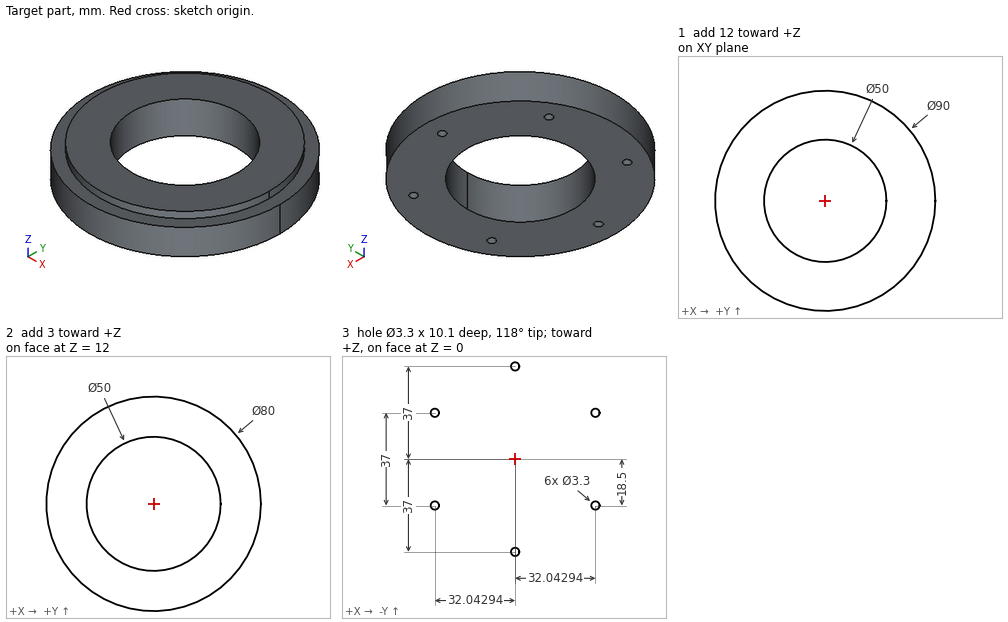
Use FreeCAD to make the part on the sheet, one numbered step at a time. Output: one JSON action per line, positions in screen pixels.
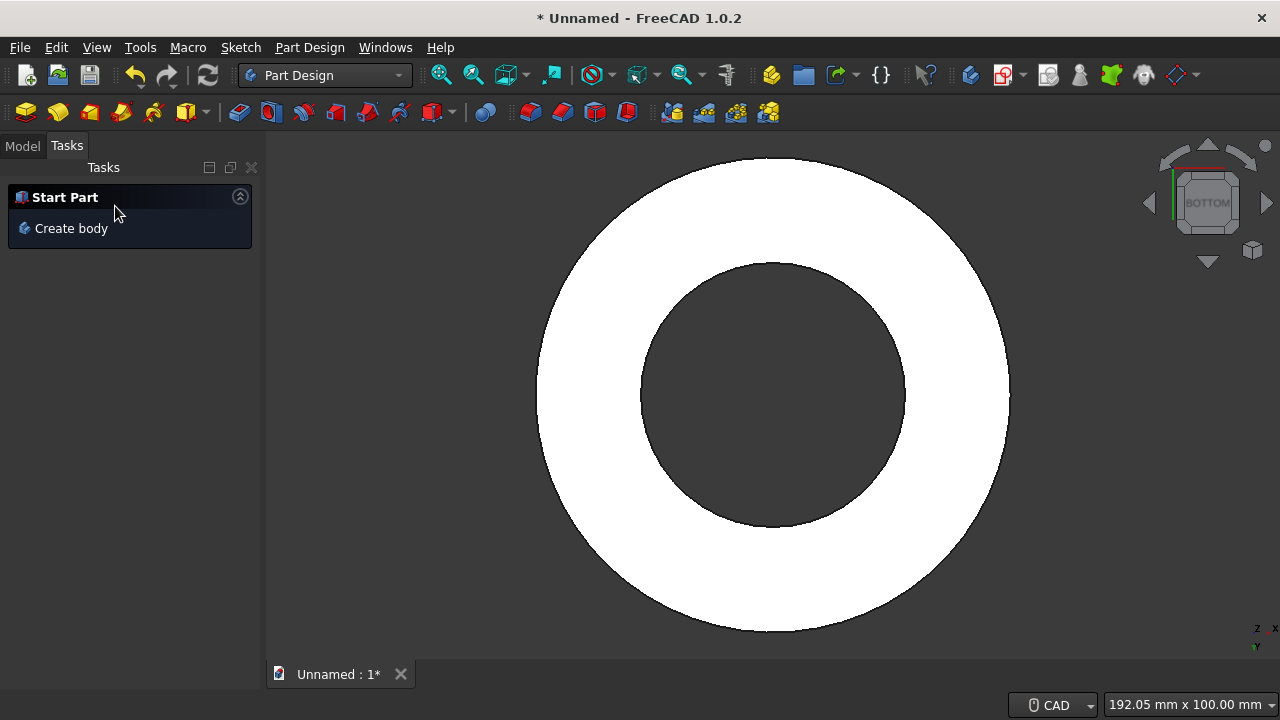
{"action": "left_click", "coordinate": [909, 530]}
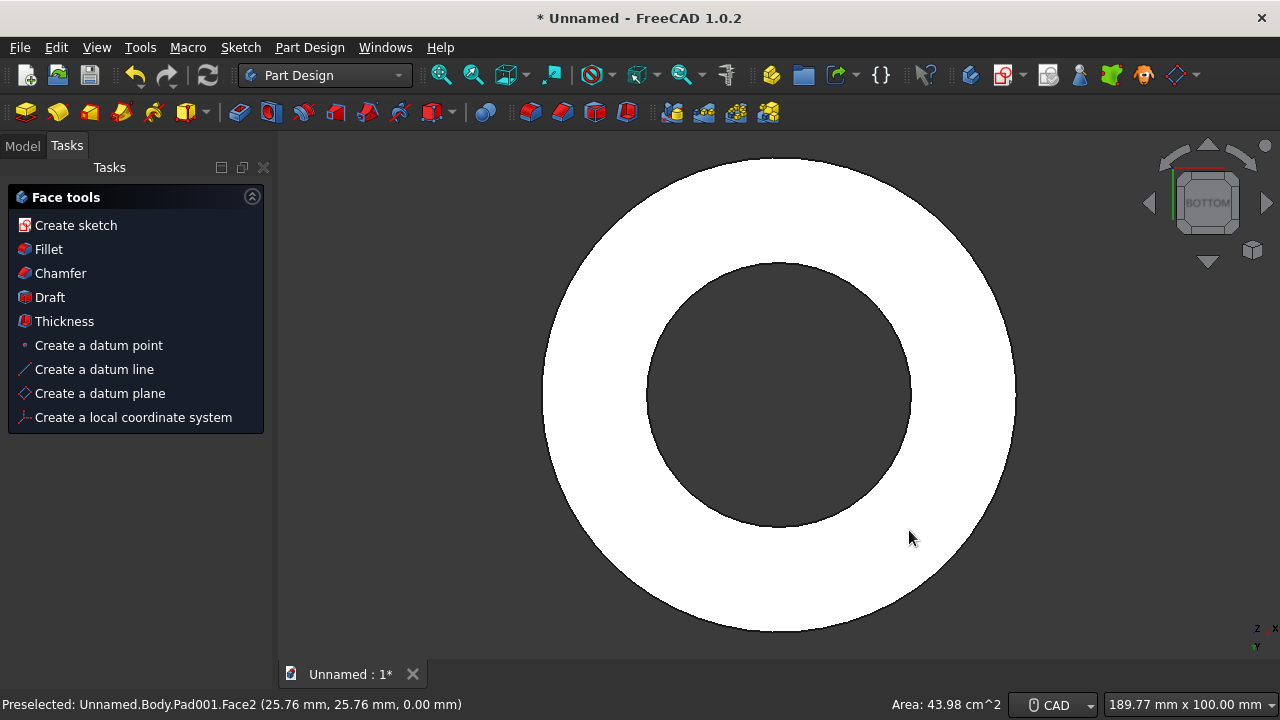
{"action": "left_click", "coordinate": [1004, 76]}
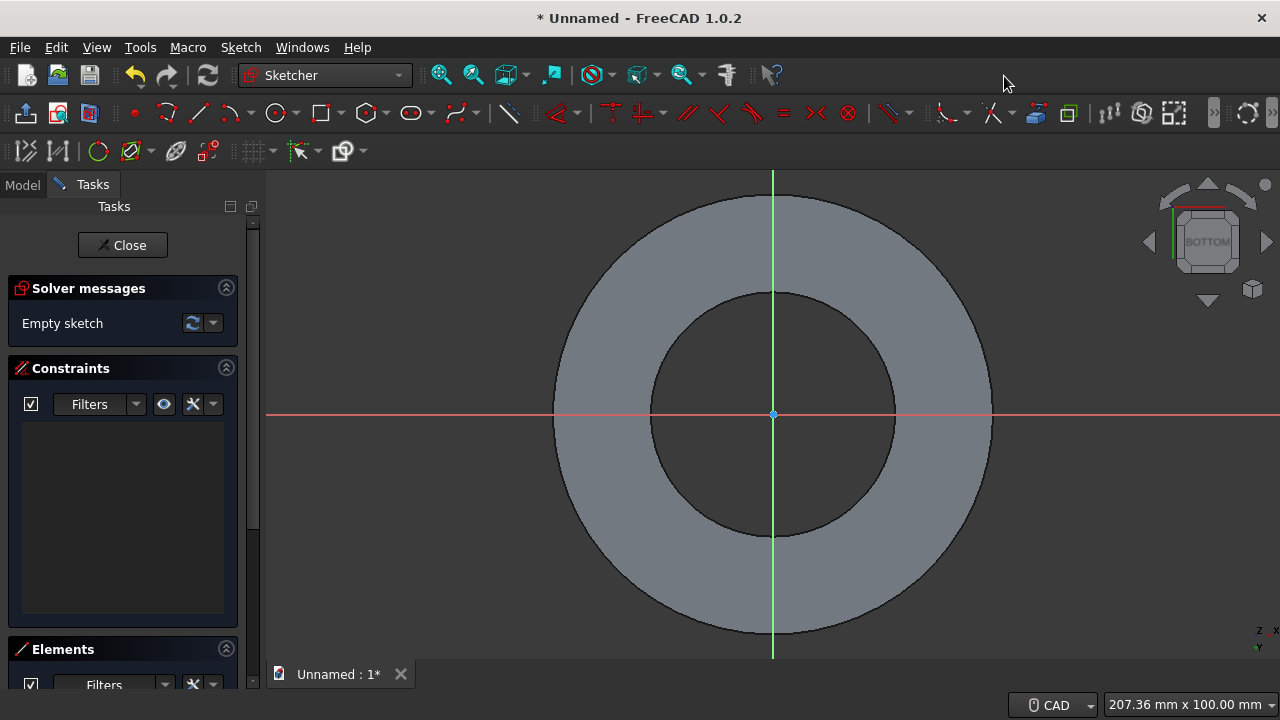
{"action": "left_click", "coordinate": [276, 114]}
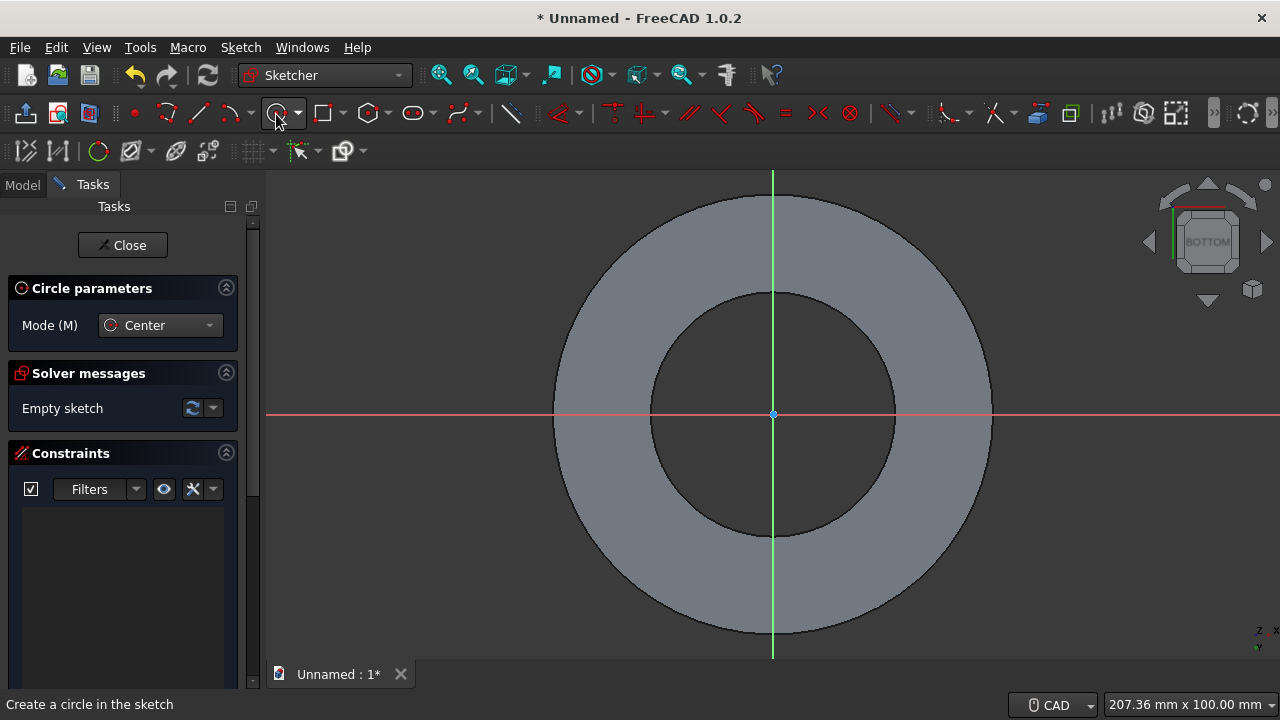
{"action": "scroll", "coordinate": [930, 505], "scroll_direction": "up", "scroll_amount": 6}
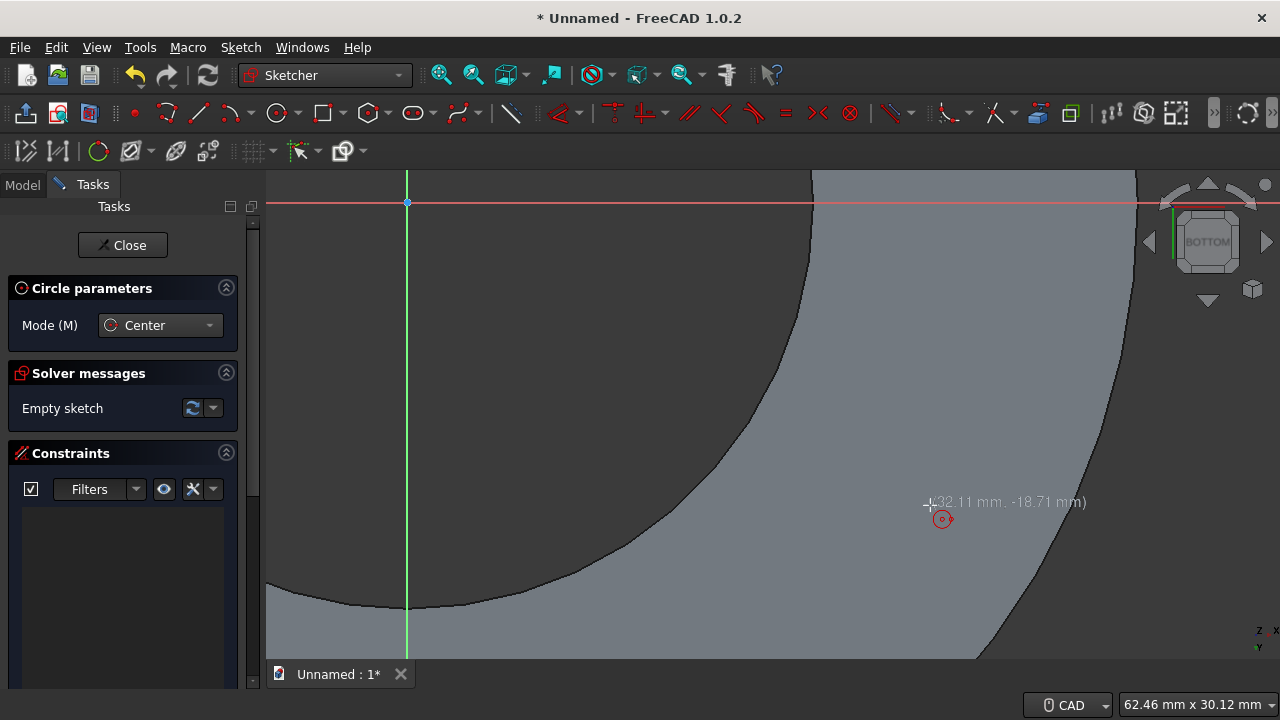
{"action": "left_click", "coordinate": [927, 503]}
{"action": "left_click", "coordinate": [946, 484]}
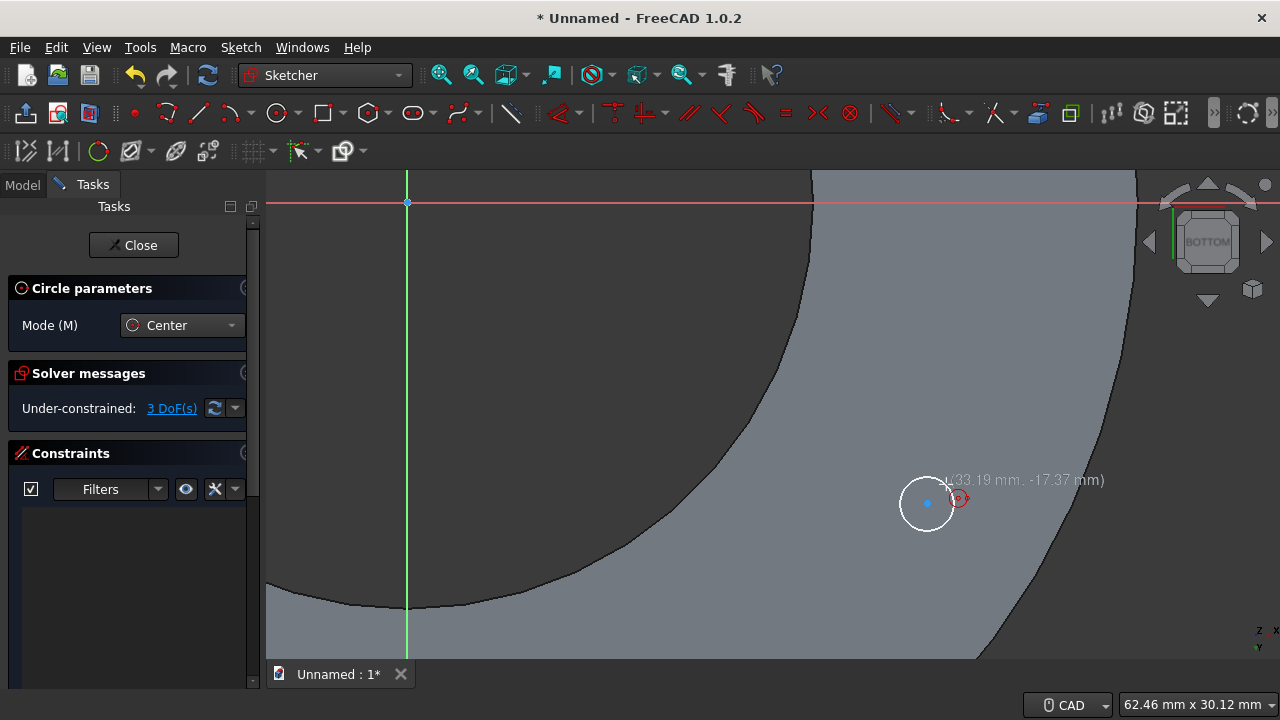
{"action": "scroll", "coordinate": [802, 484], "scroll_direction": "down", "scroll_amount": 7}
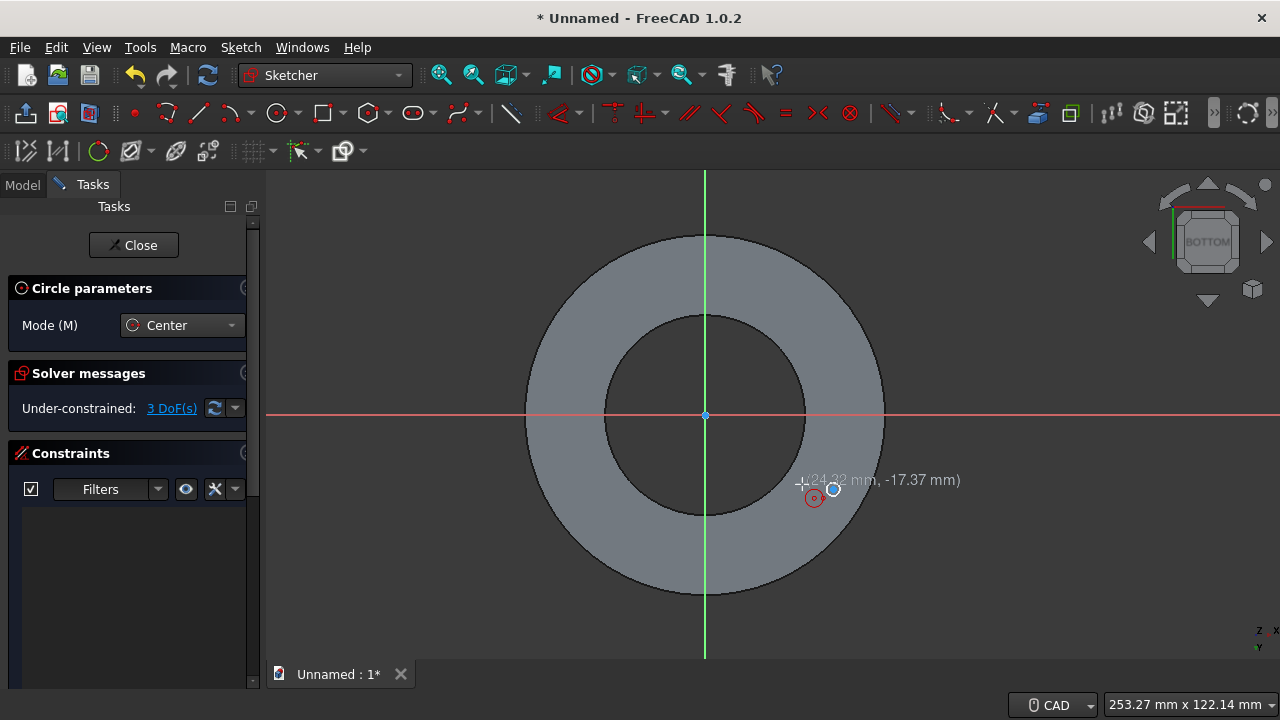
{"action": "scroll", "coordinate": [705, 563], "scroll_direction": "up", "scroll_amount": 7}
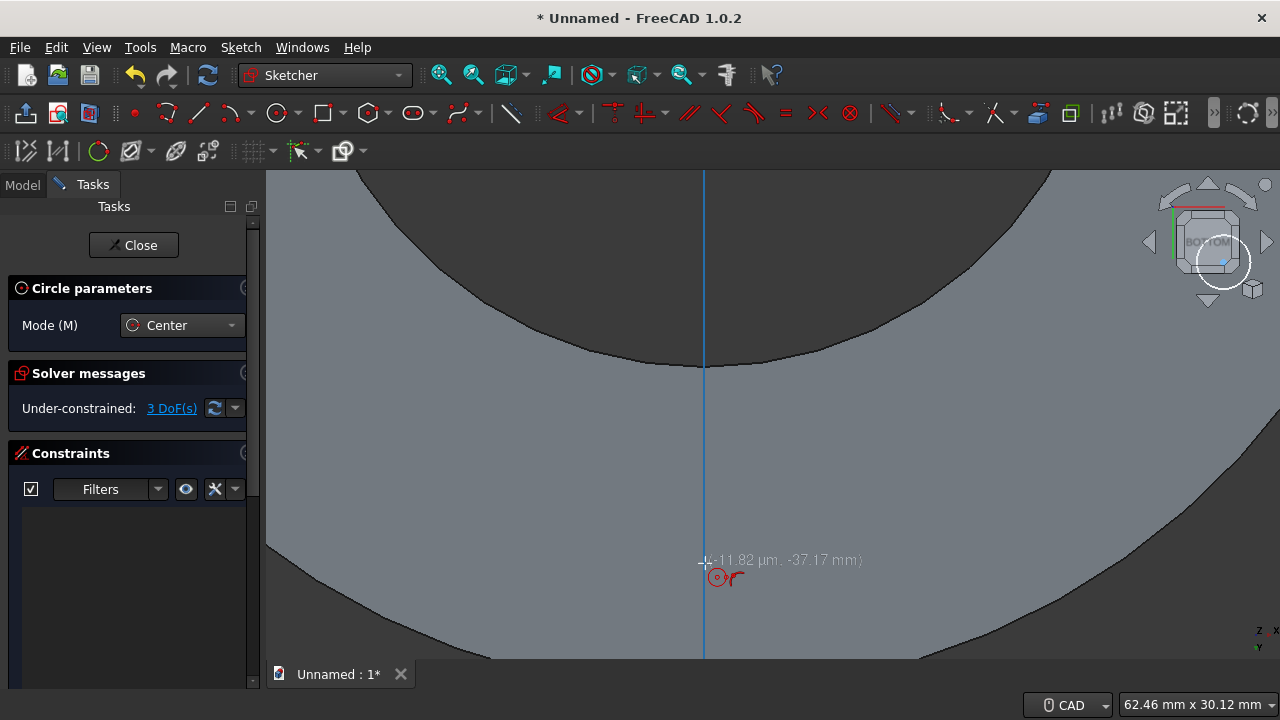
{"action": "left_click", "coordinate": [704, 562]}
{"action": "left_click", "coordinate": [723, 543]}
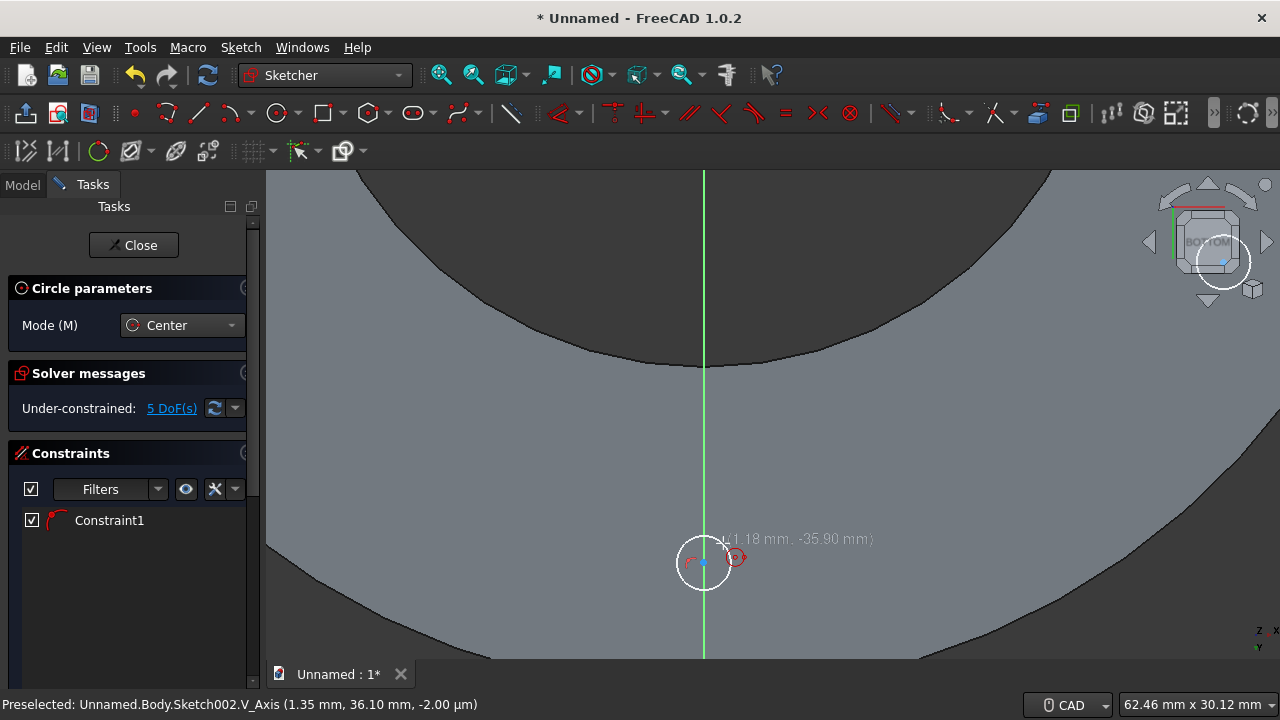
{"action": "scroll", "coordinate": [705, 563], "scroll_direction": "down", "scroll_amount": 7}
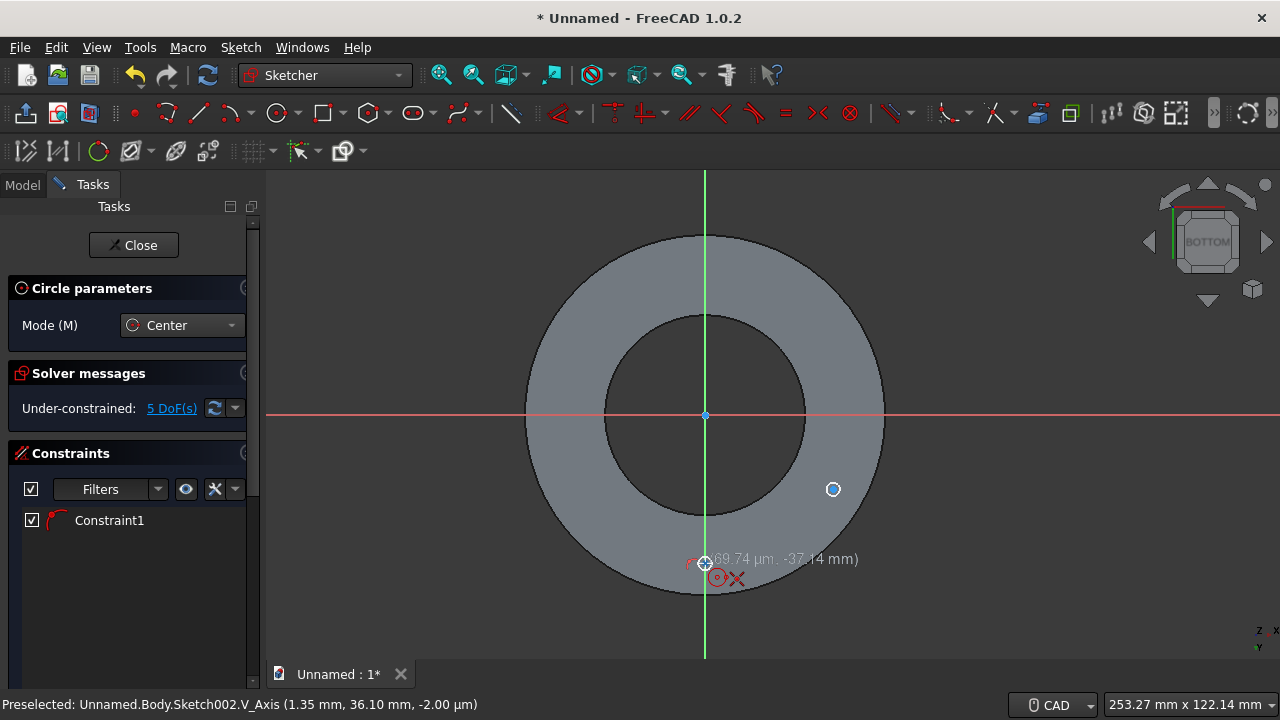
{"action": "scroll", "coordinate": [577, 489], "scroll_direction": "up", "scroll_amount": 7}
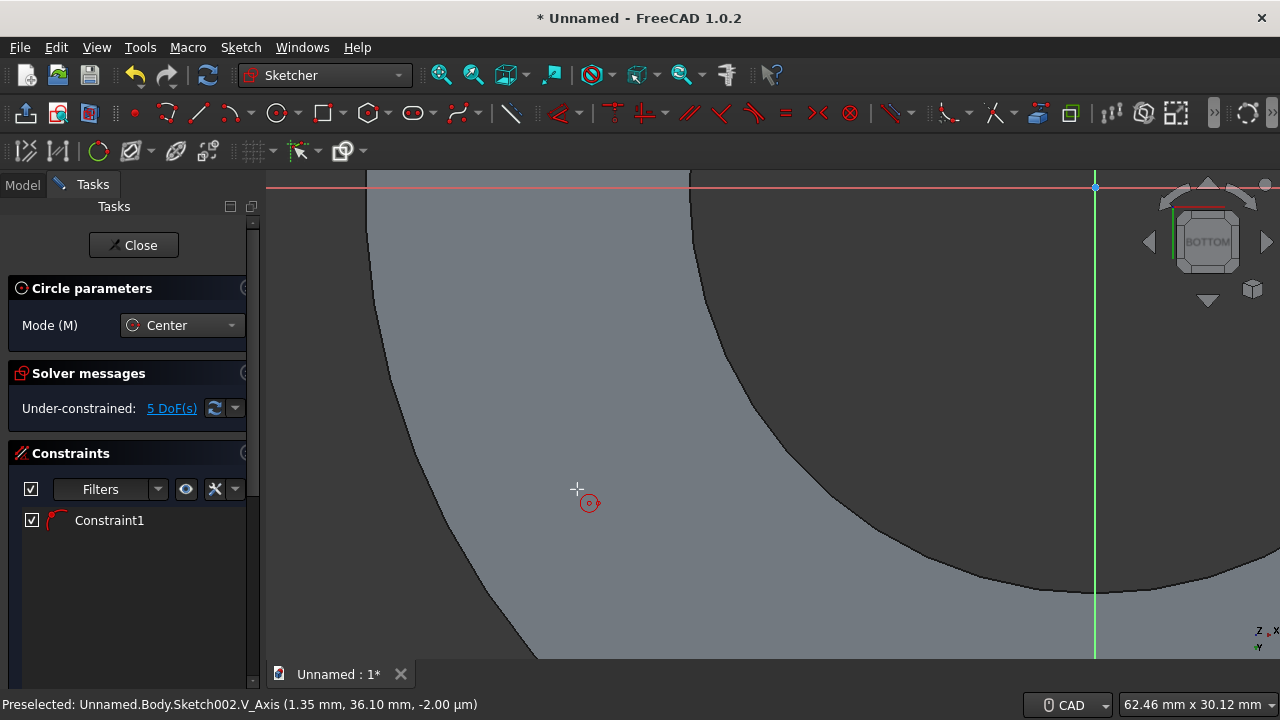
{"action": "left_click", "coordinate": [575, 488]}
{"action": "left_click", "coordinate": [594, 469]}